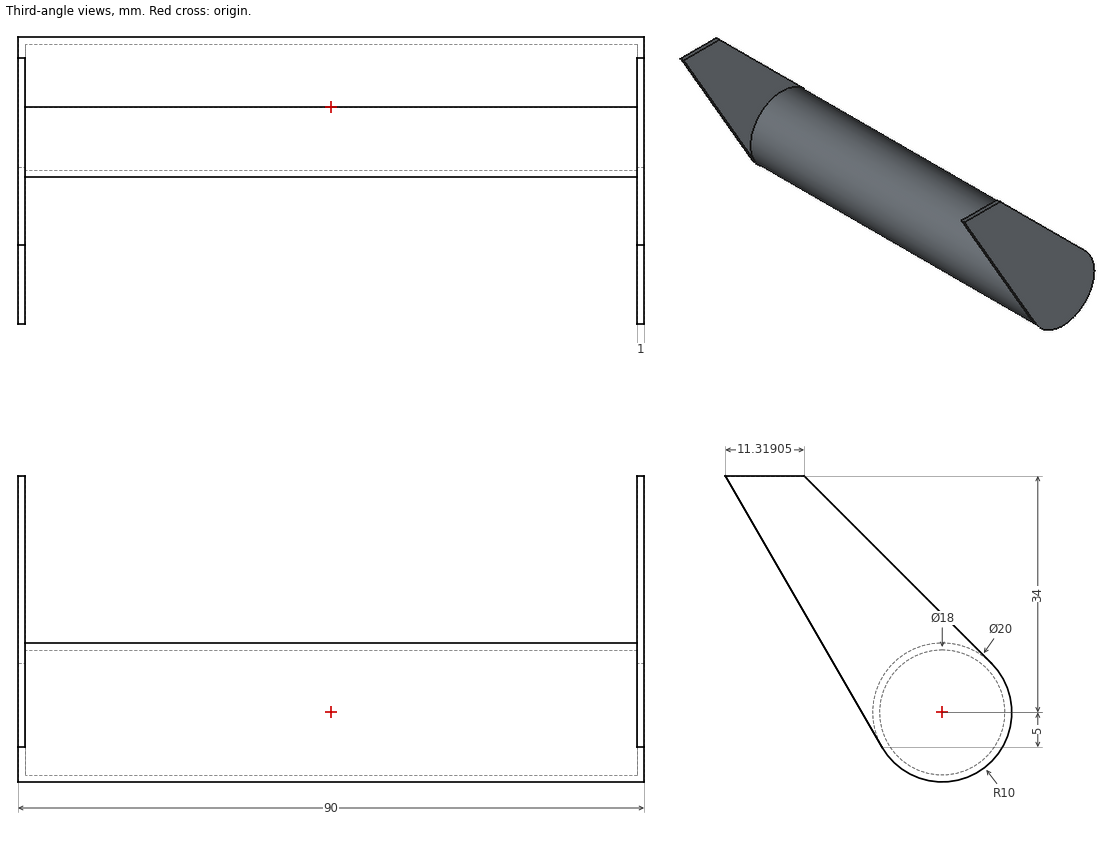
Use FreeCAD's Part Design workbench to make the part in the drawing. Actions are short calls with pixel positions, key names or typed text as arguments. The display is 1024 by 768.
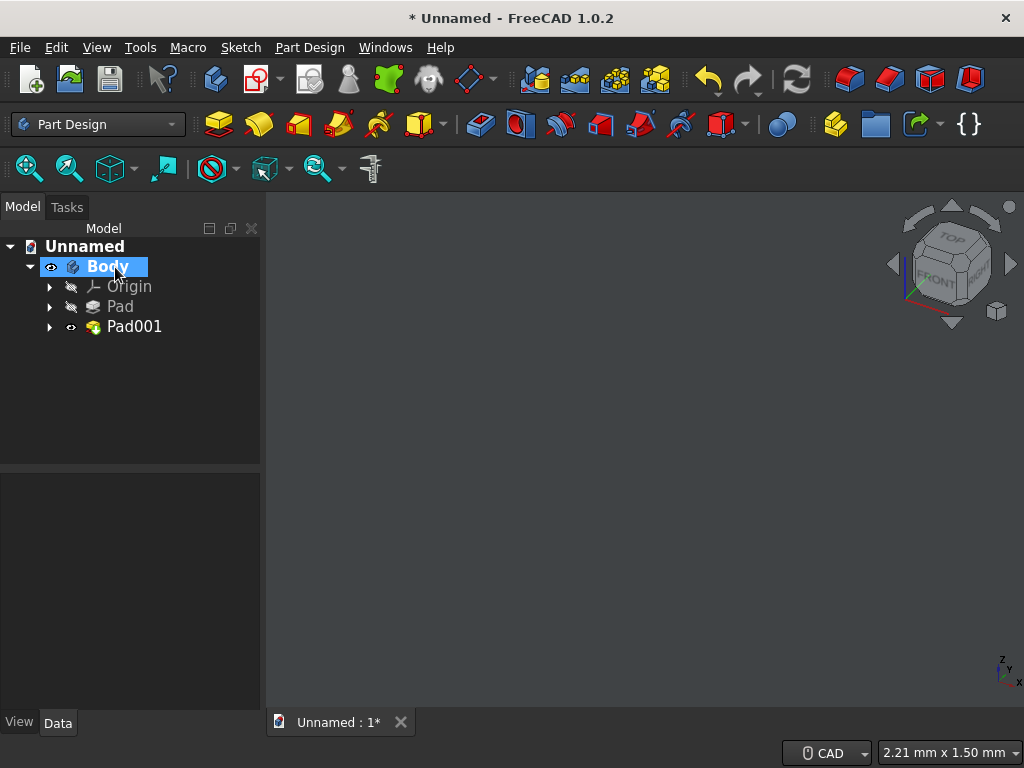
key(v)
key(f)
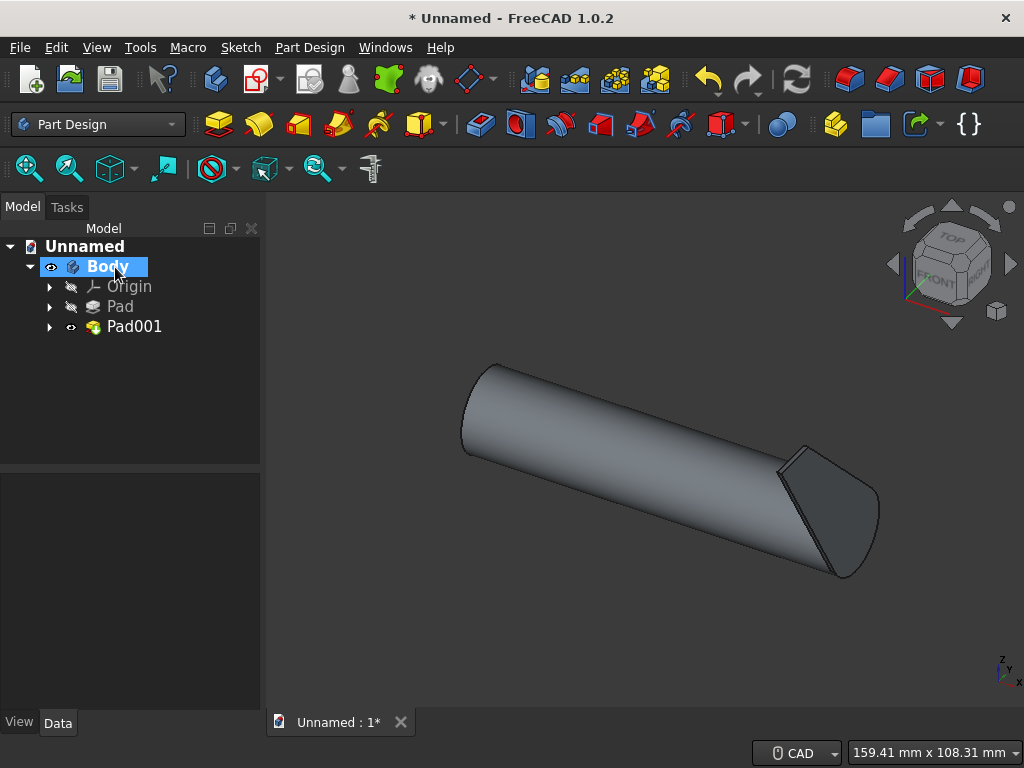
click(116, 327)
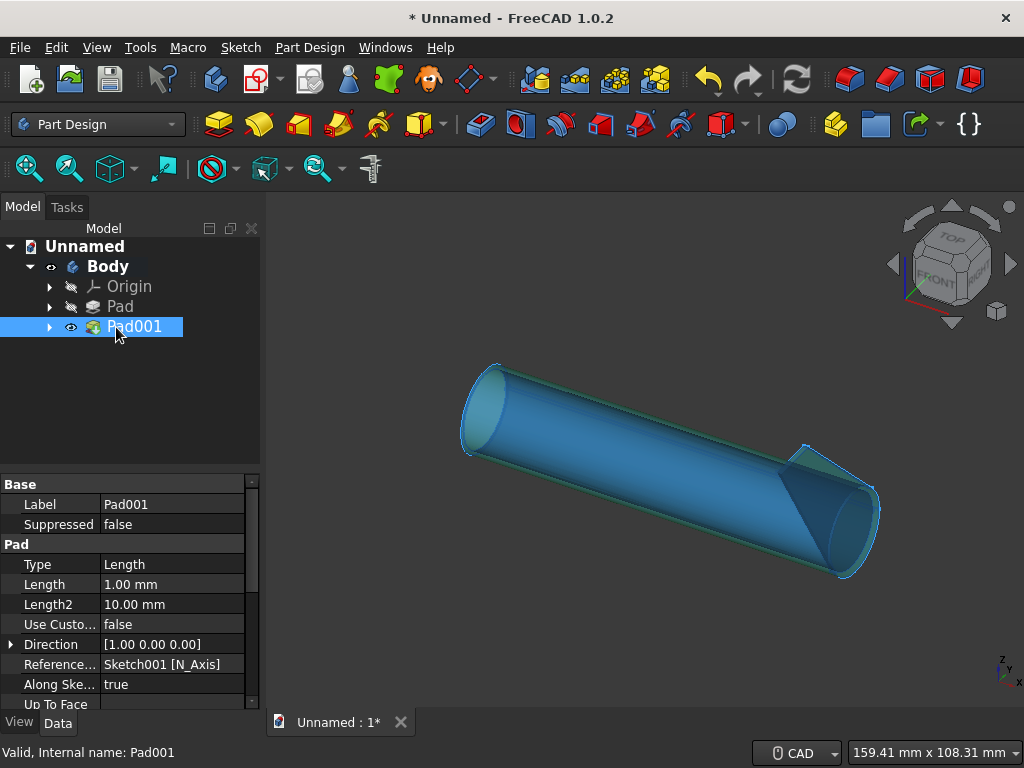
click(536, 80)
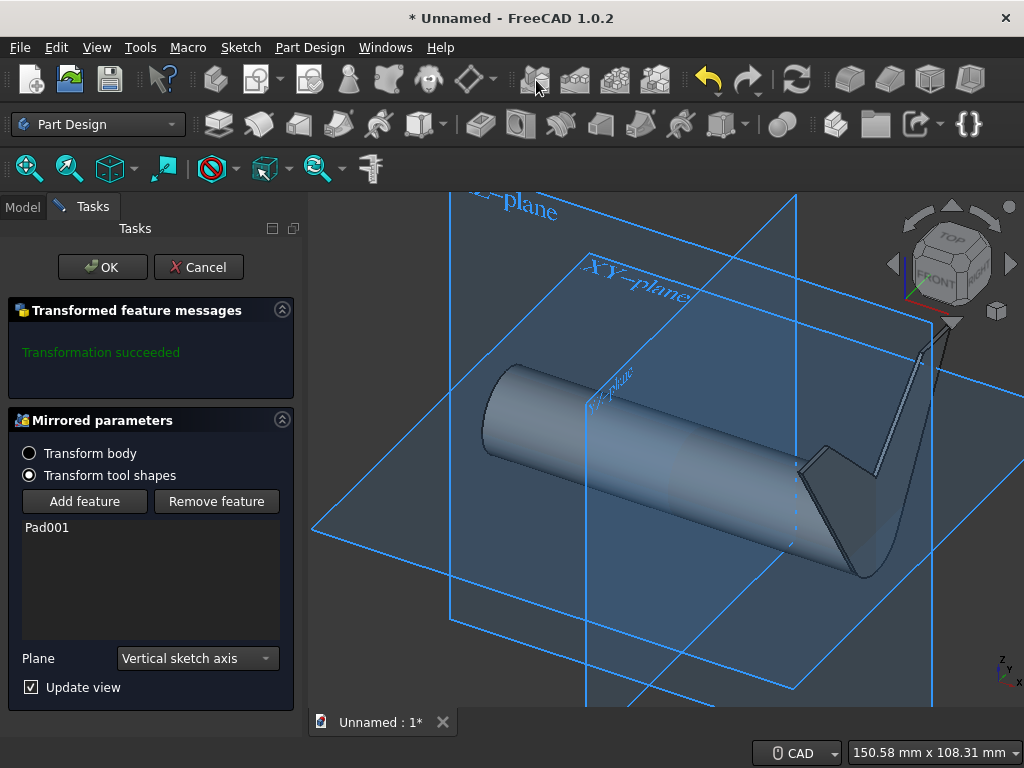
click(198, 658)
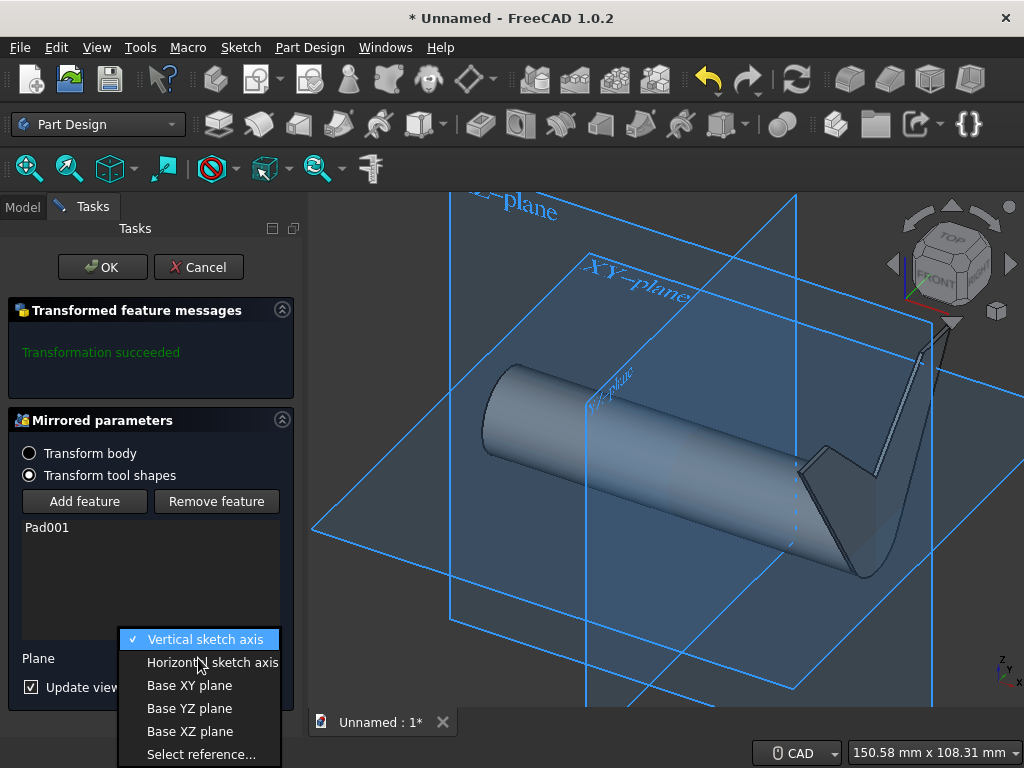
click(198, 708)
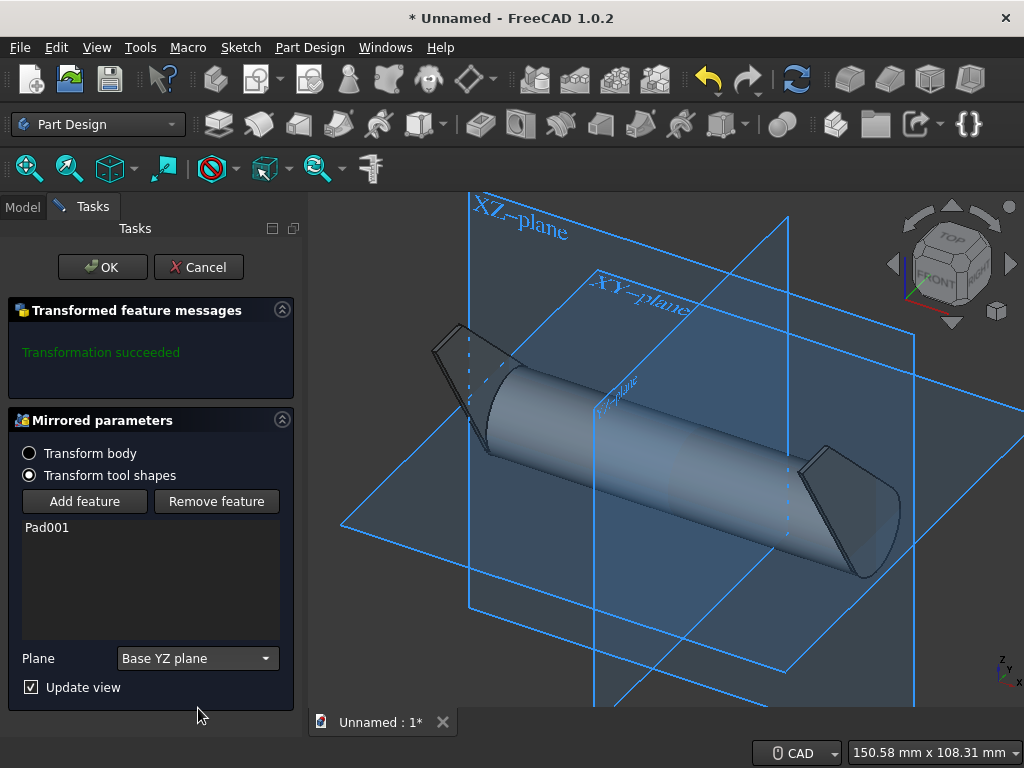
click(103, 267)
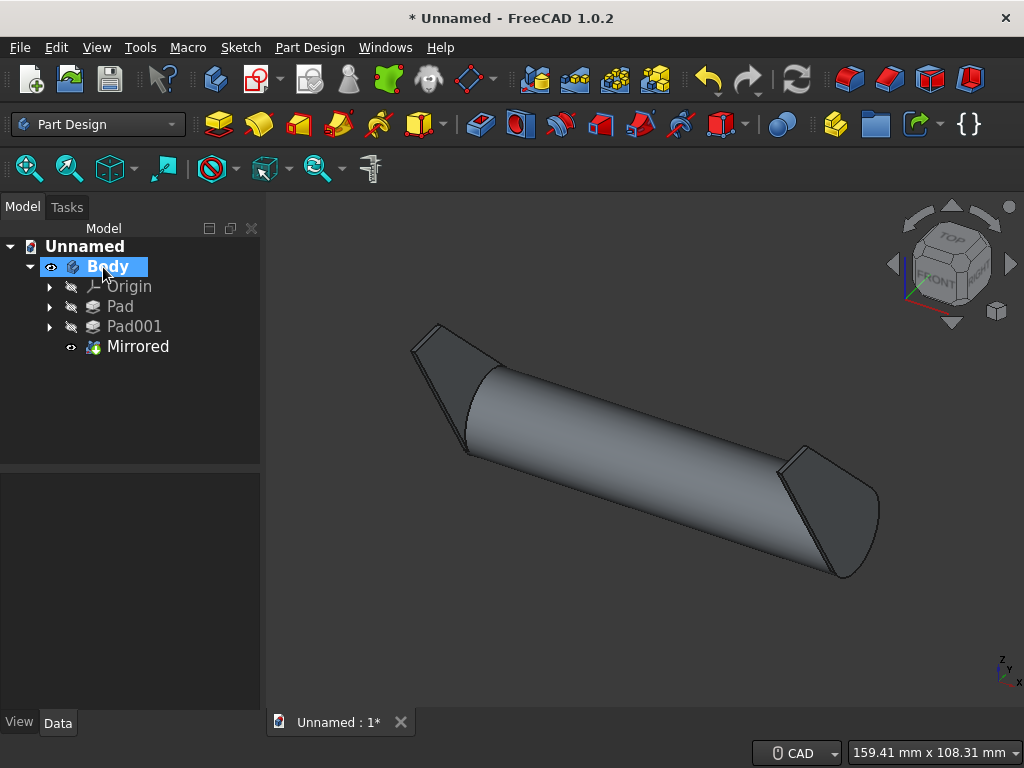
key(0)